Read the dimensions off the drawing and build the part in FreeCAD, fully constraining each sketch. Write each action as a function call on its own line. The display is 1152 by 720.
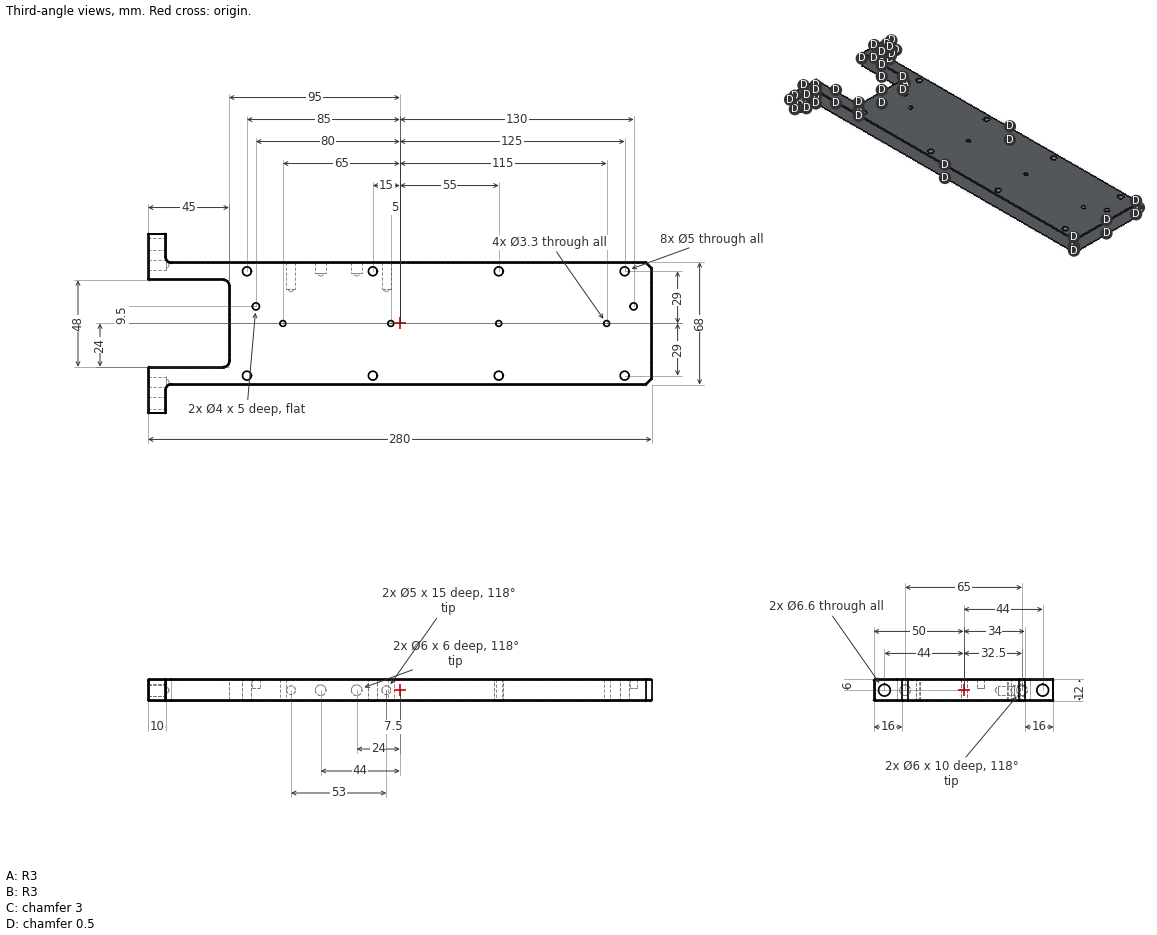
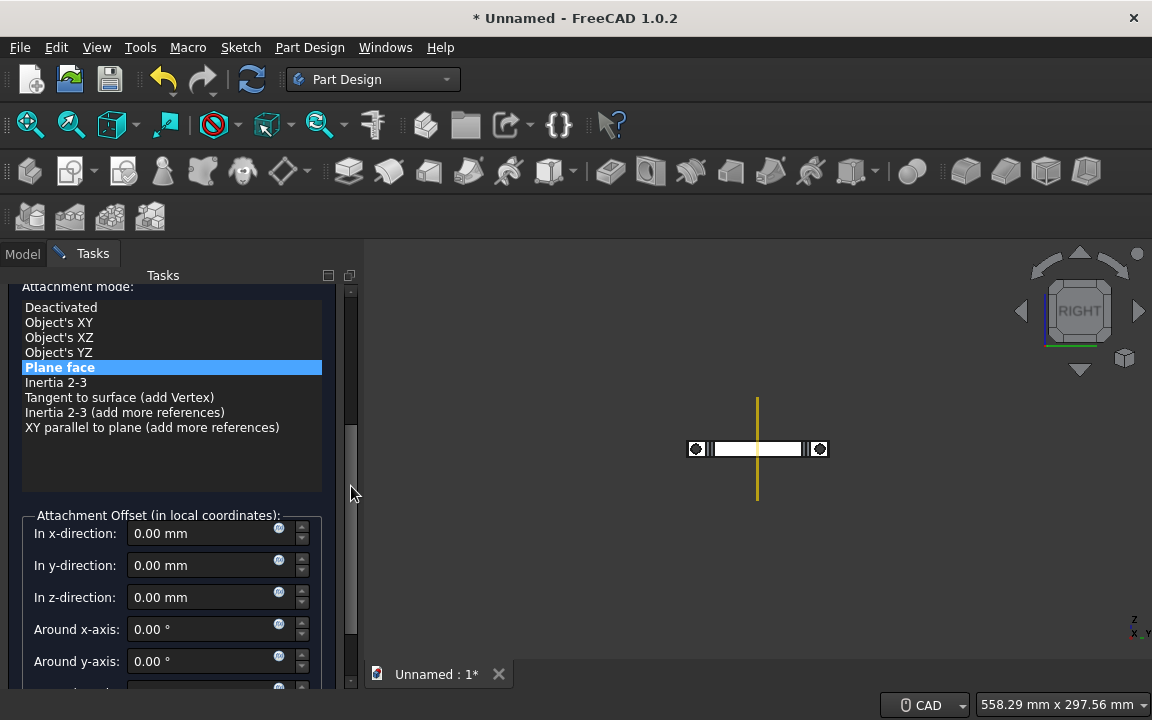
triple_click(210, 597)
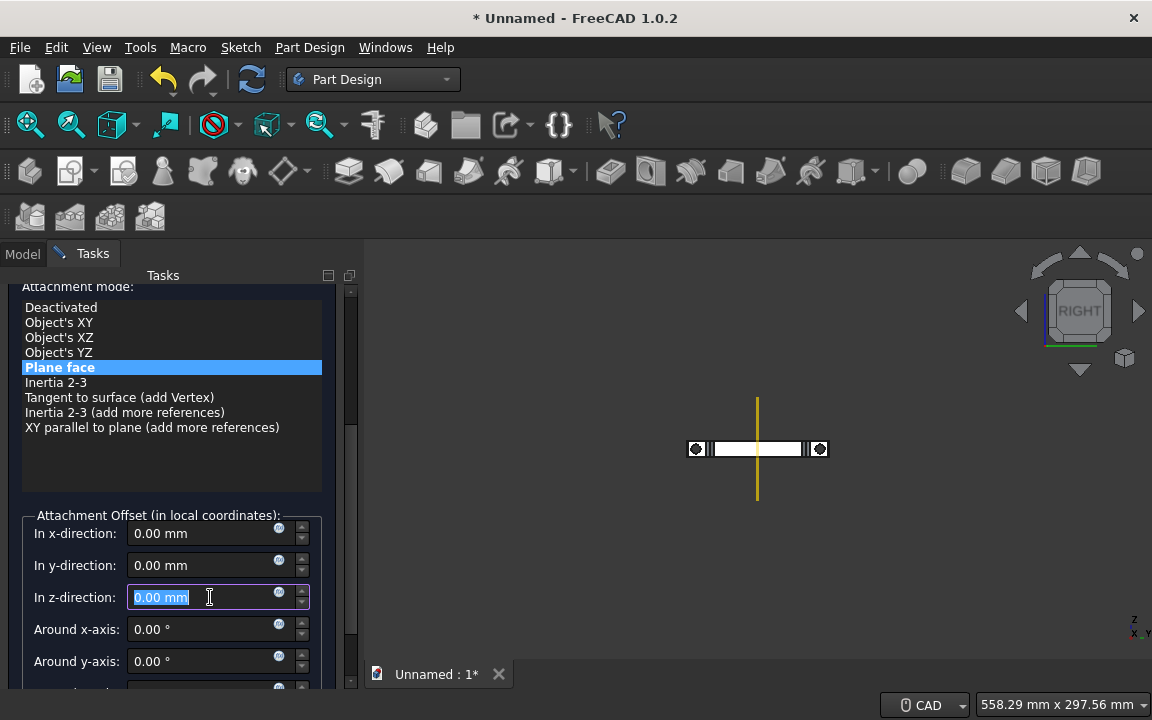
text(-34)
key(Tab)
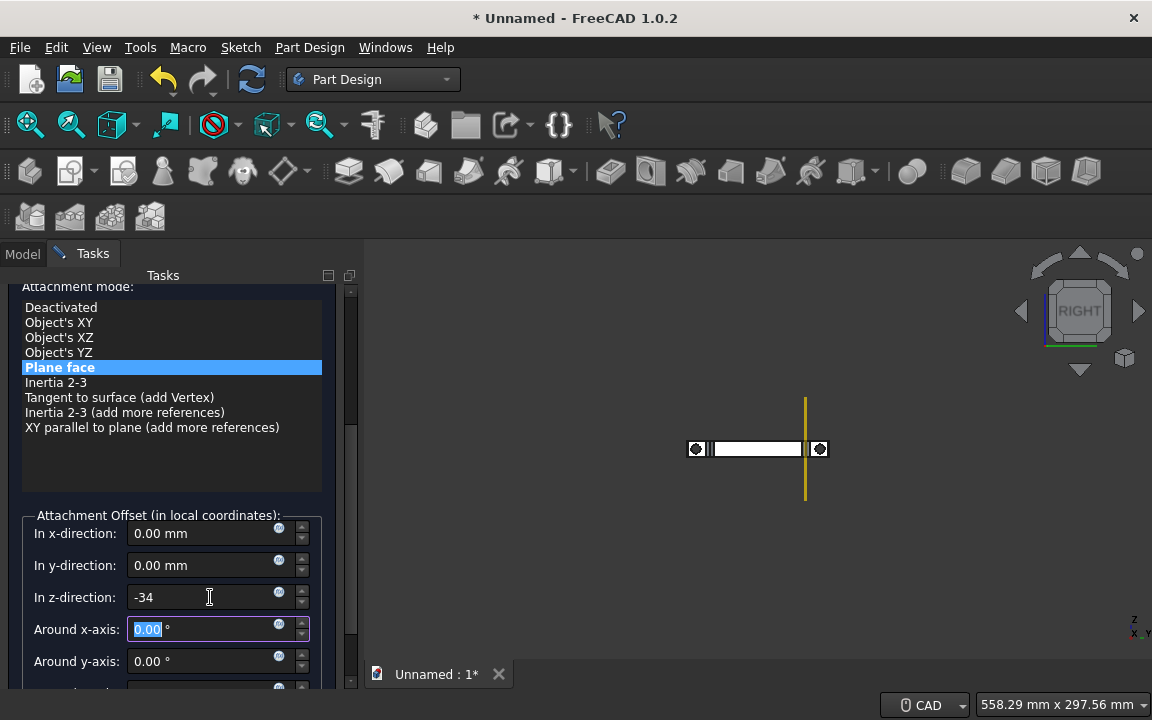
scroll(351, 486, up, 5)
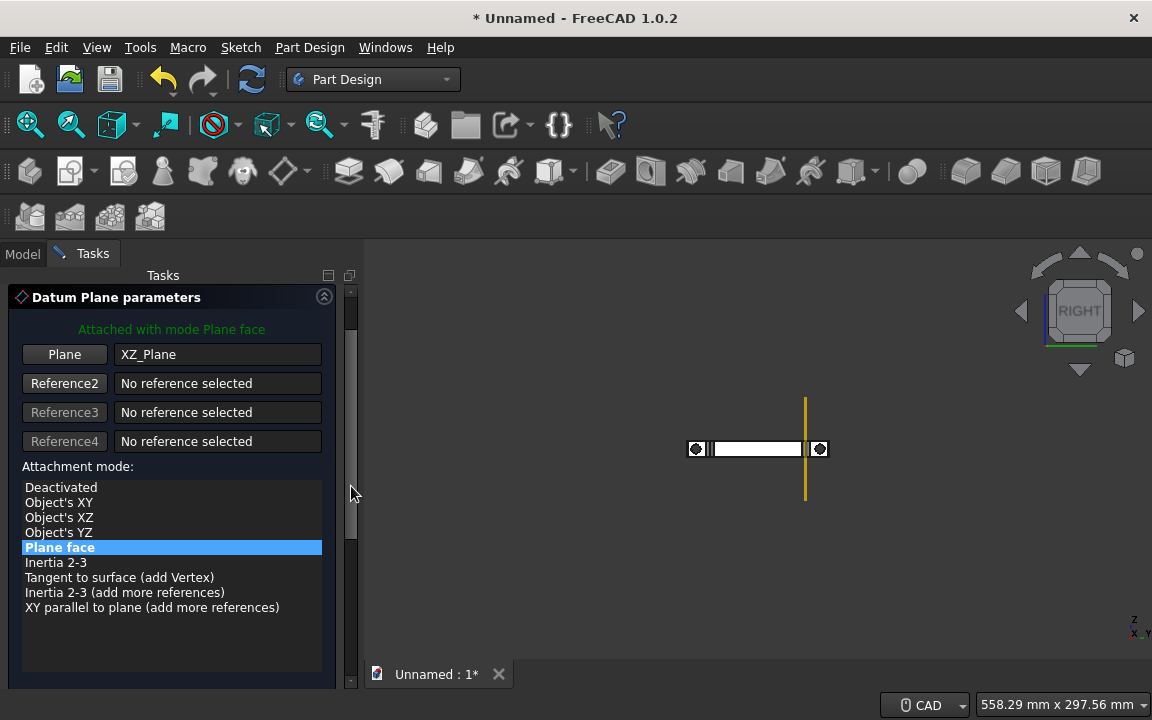
click(124, 314)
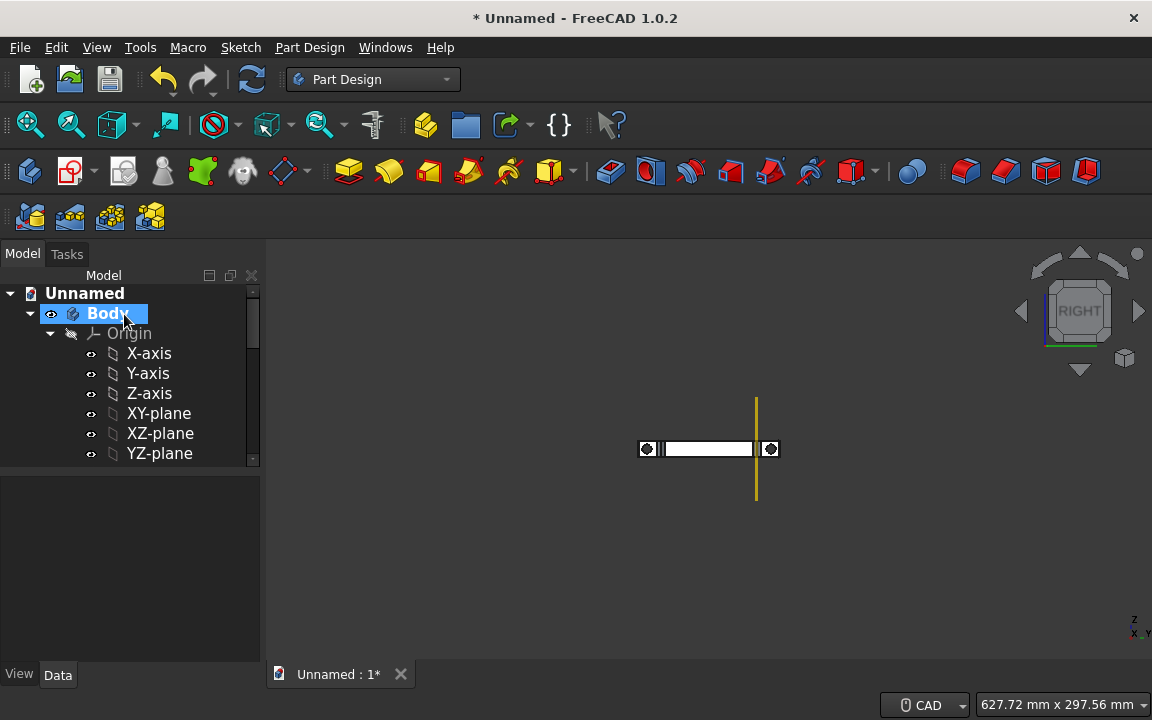
scroll(100, 369, down, 3)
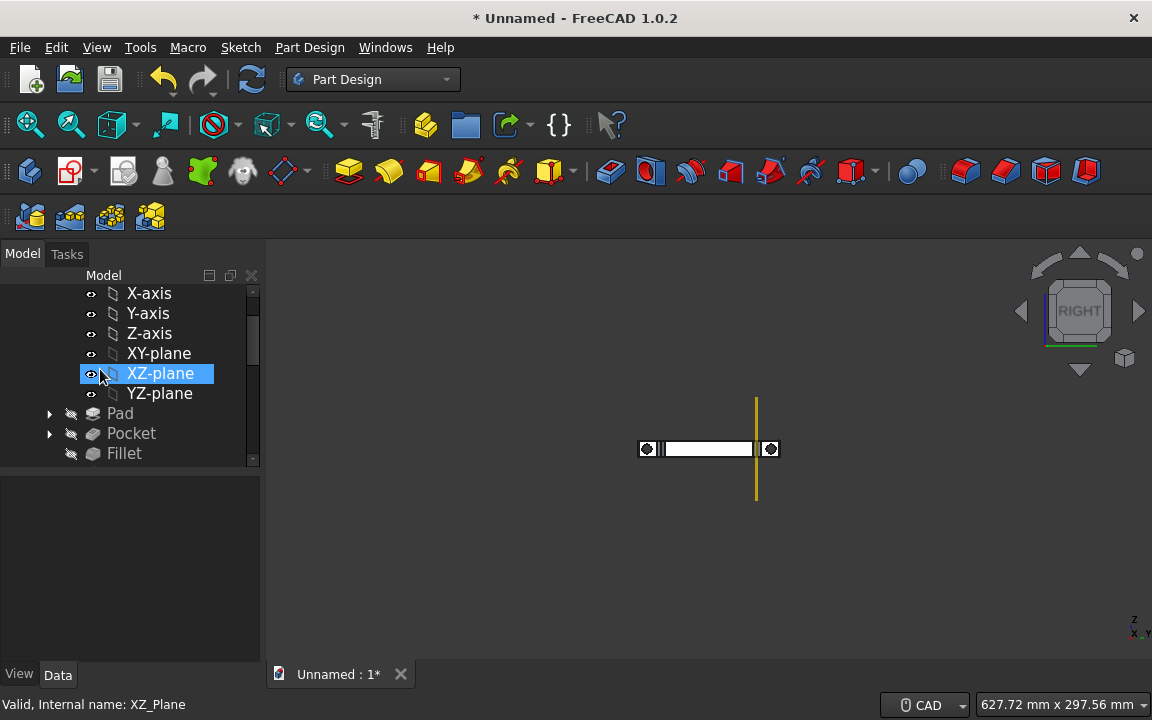
scroll(140, 369, up, 15)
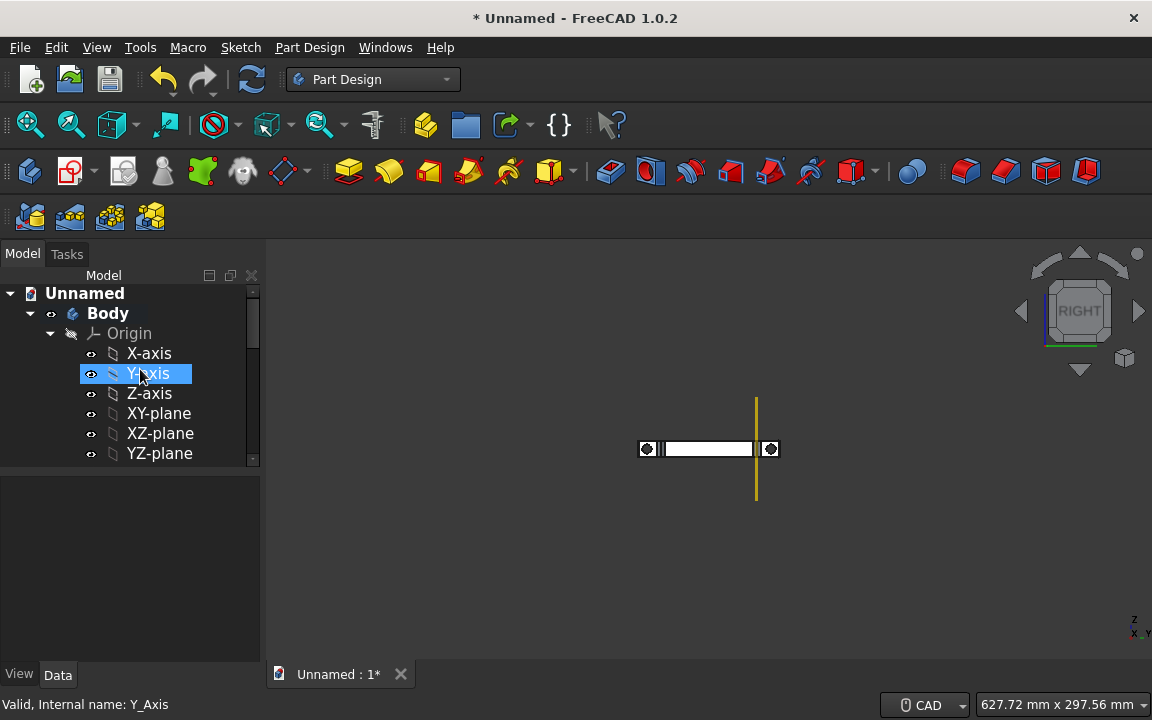
scroll(100, 369, down, 6)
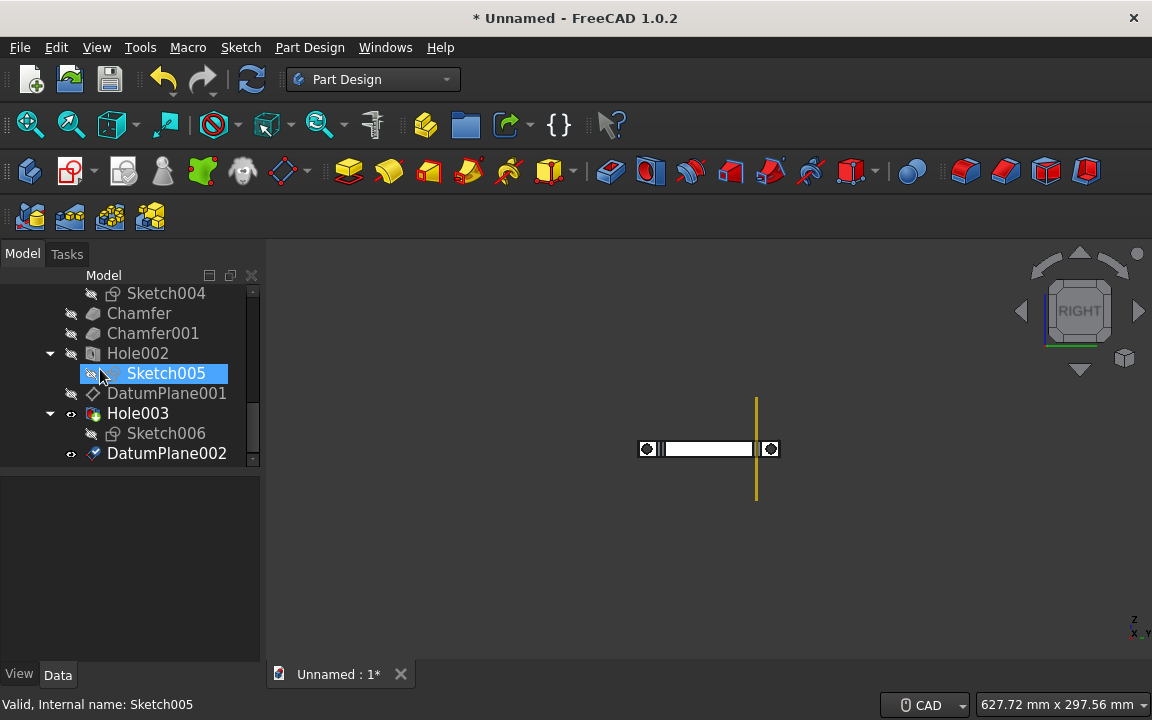
click(116, 454)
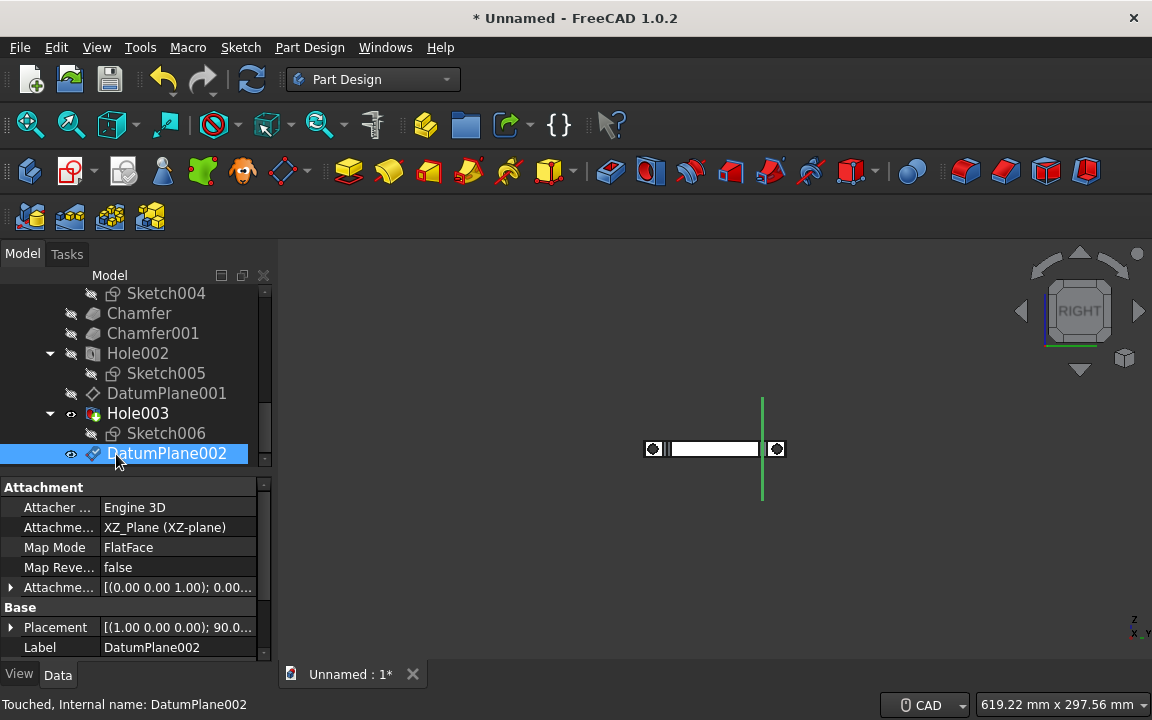
click(70, 172)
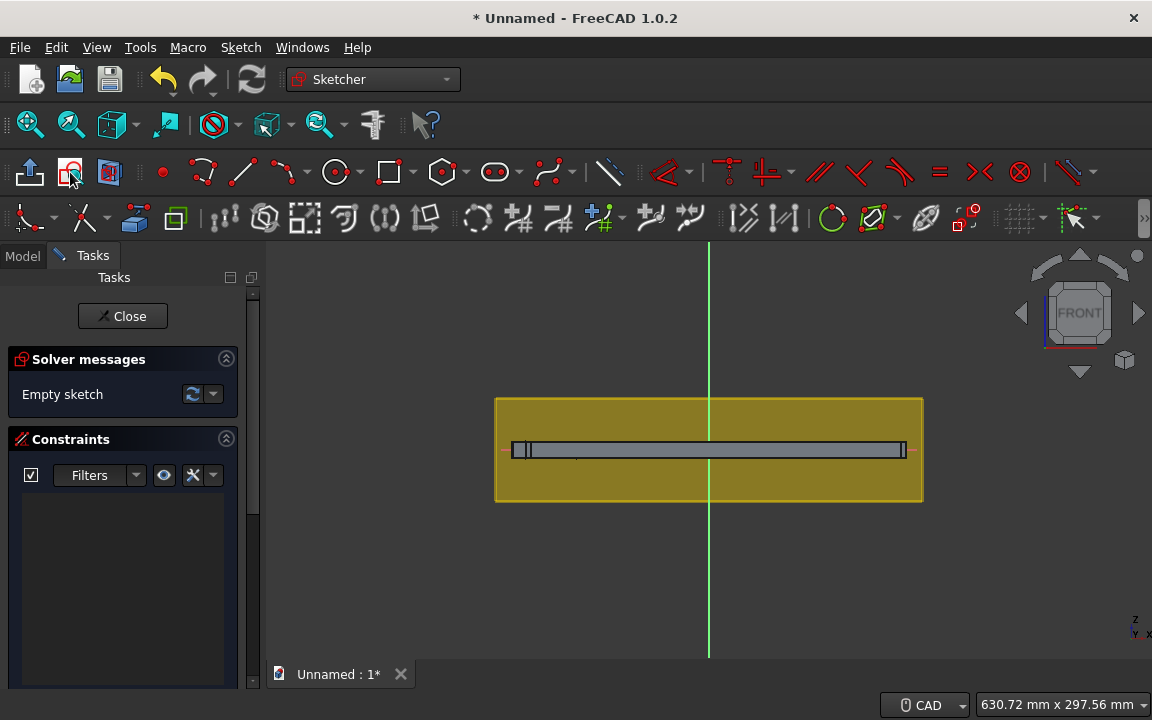
key(q)
key(s)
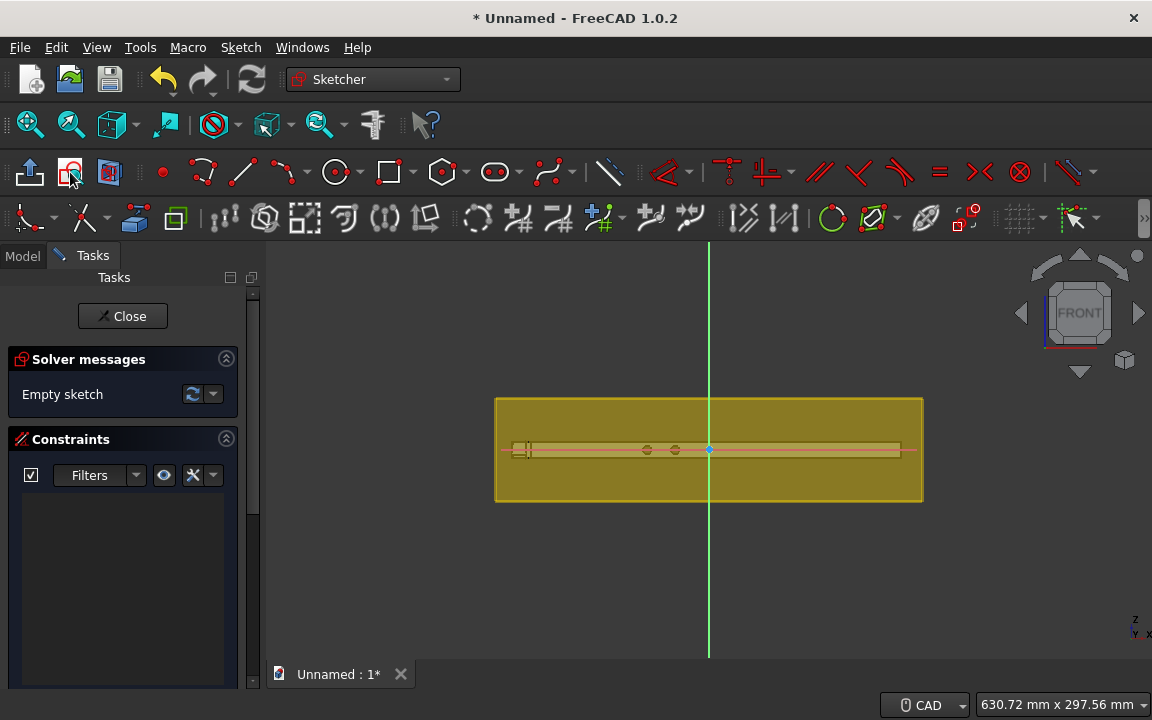
scroll(670, 450, up, 9)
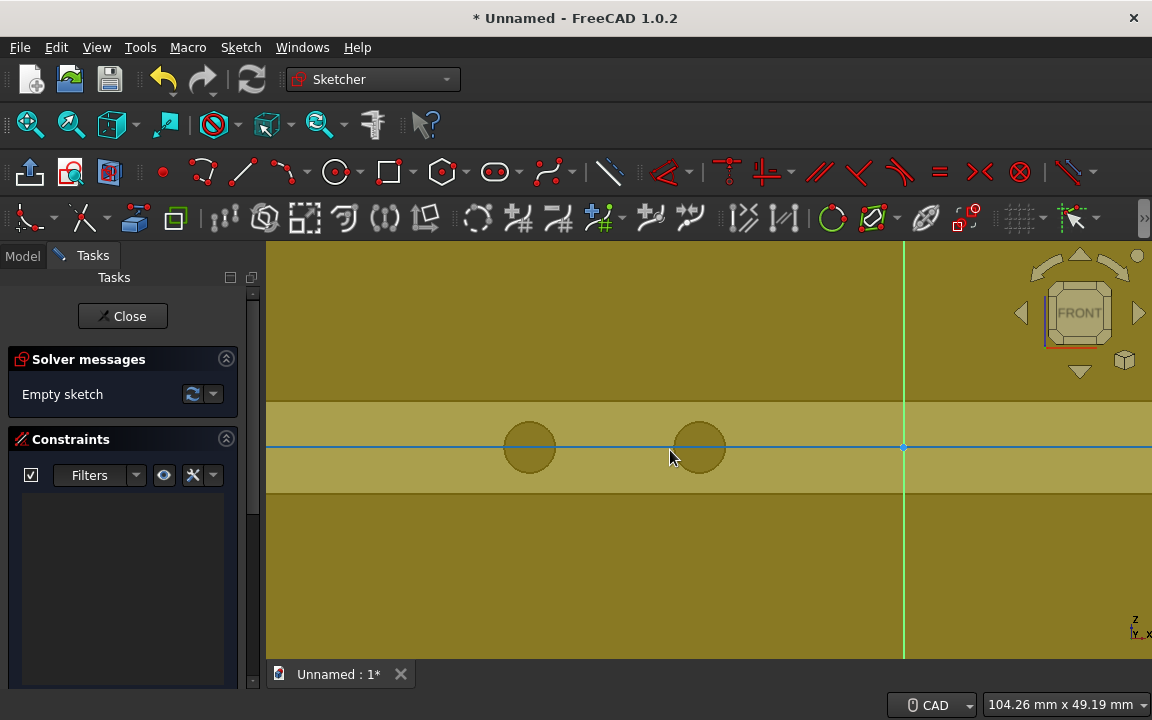
key(g)
key(c)